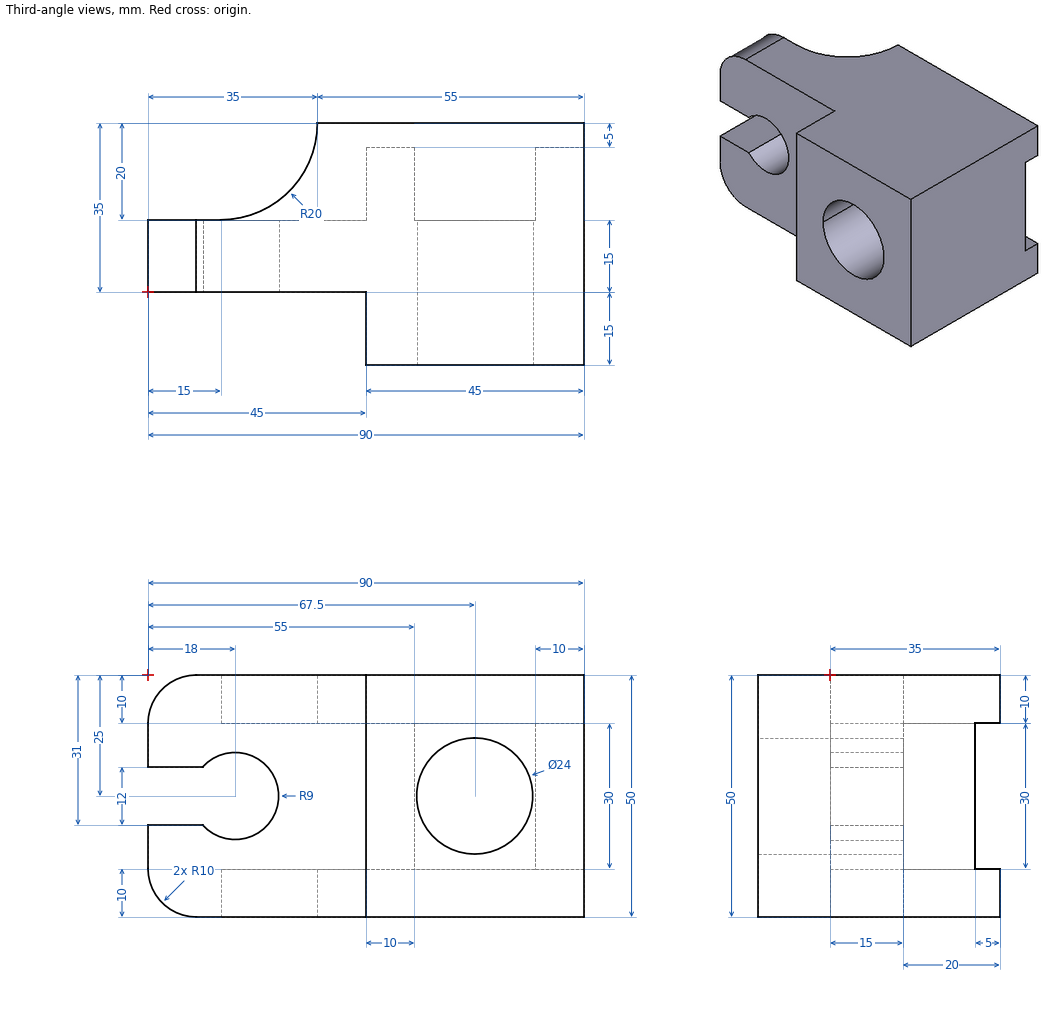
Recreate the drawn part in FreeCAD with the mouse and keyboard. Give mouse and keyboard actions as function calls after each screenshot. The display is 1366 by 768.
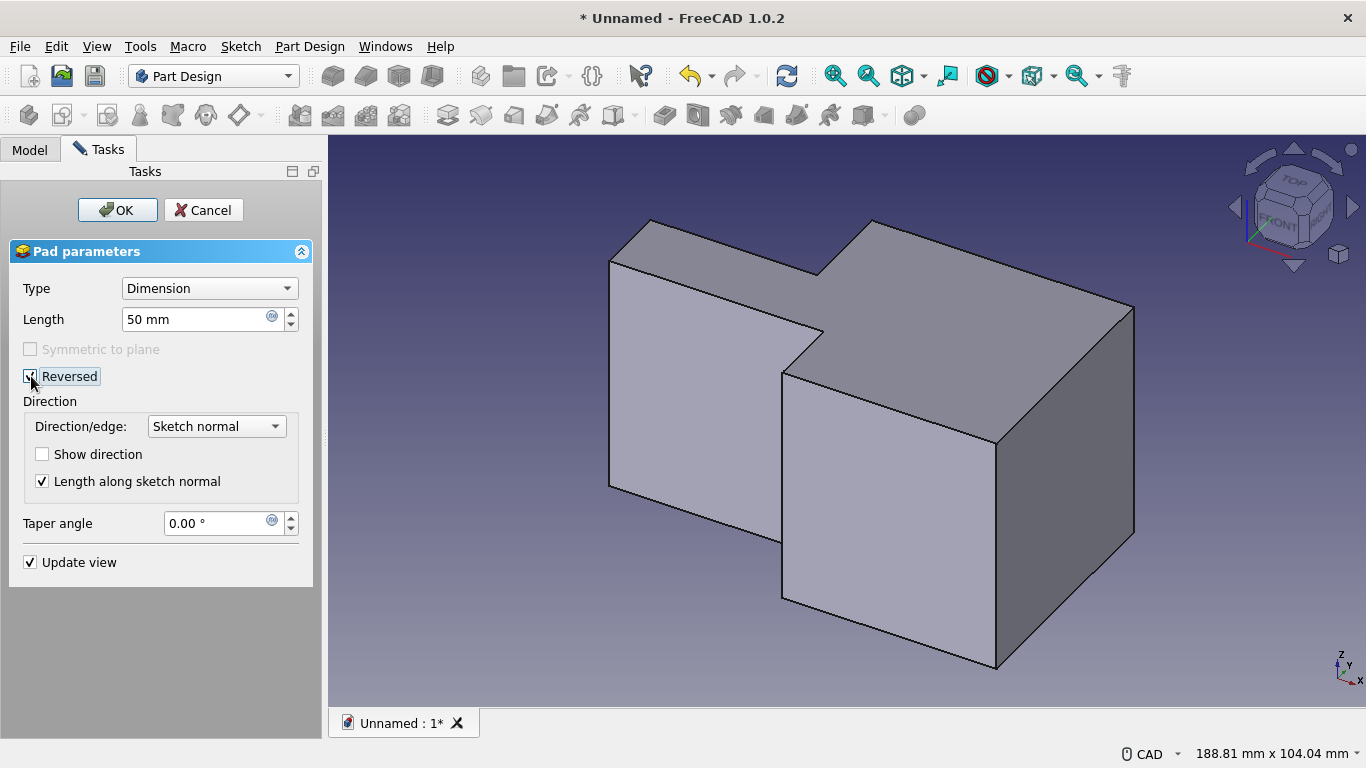
click(118, 210)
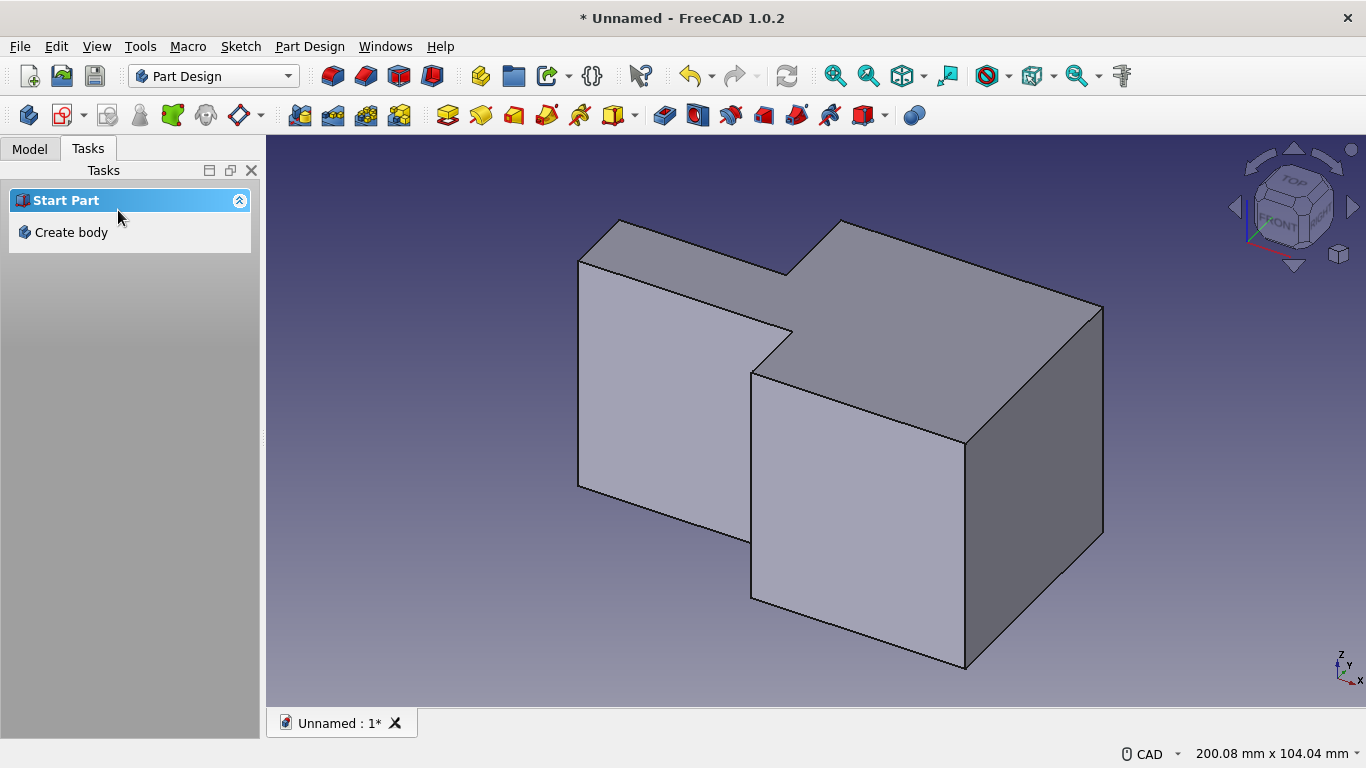
key(4)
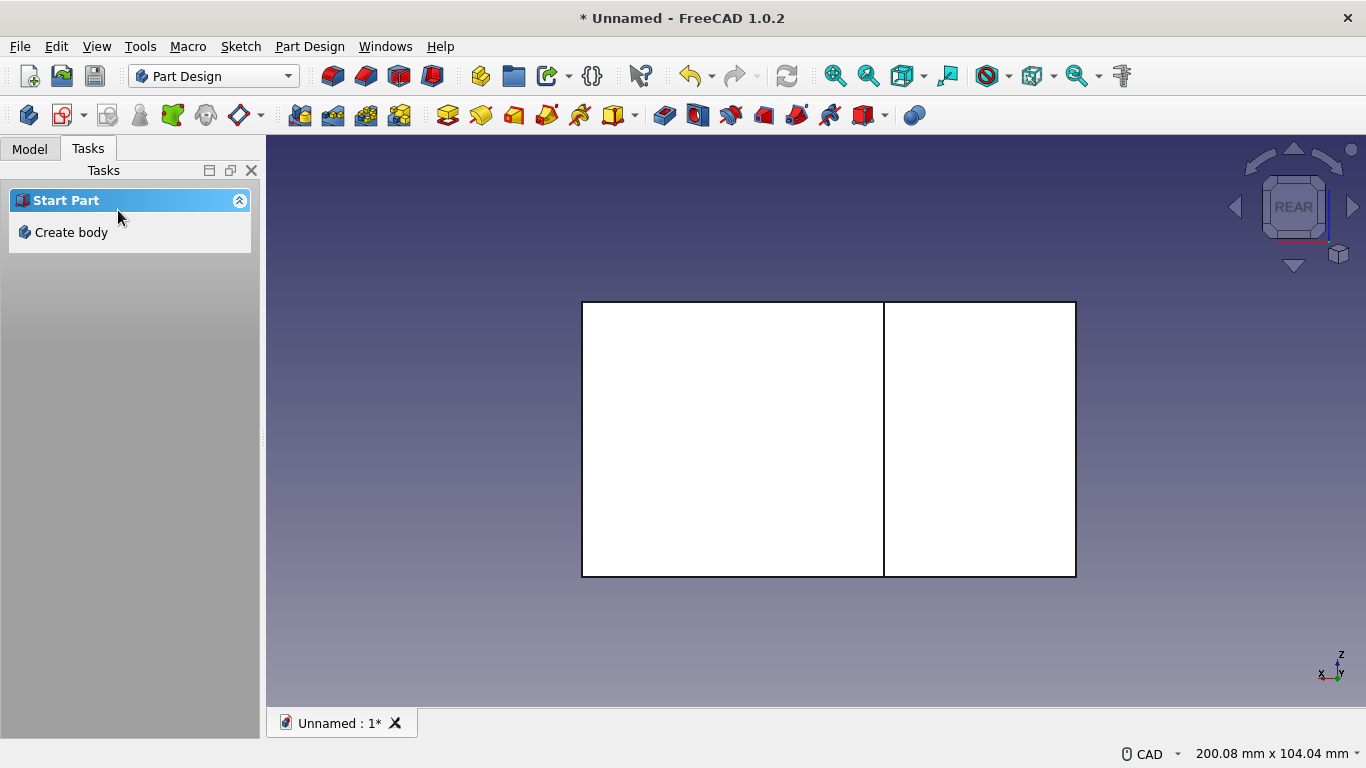
click(980, 399)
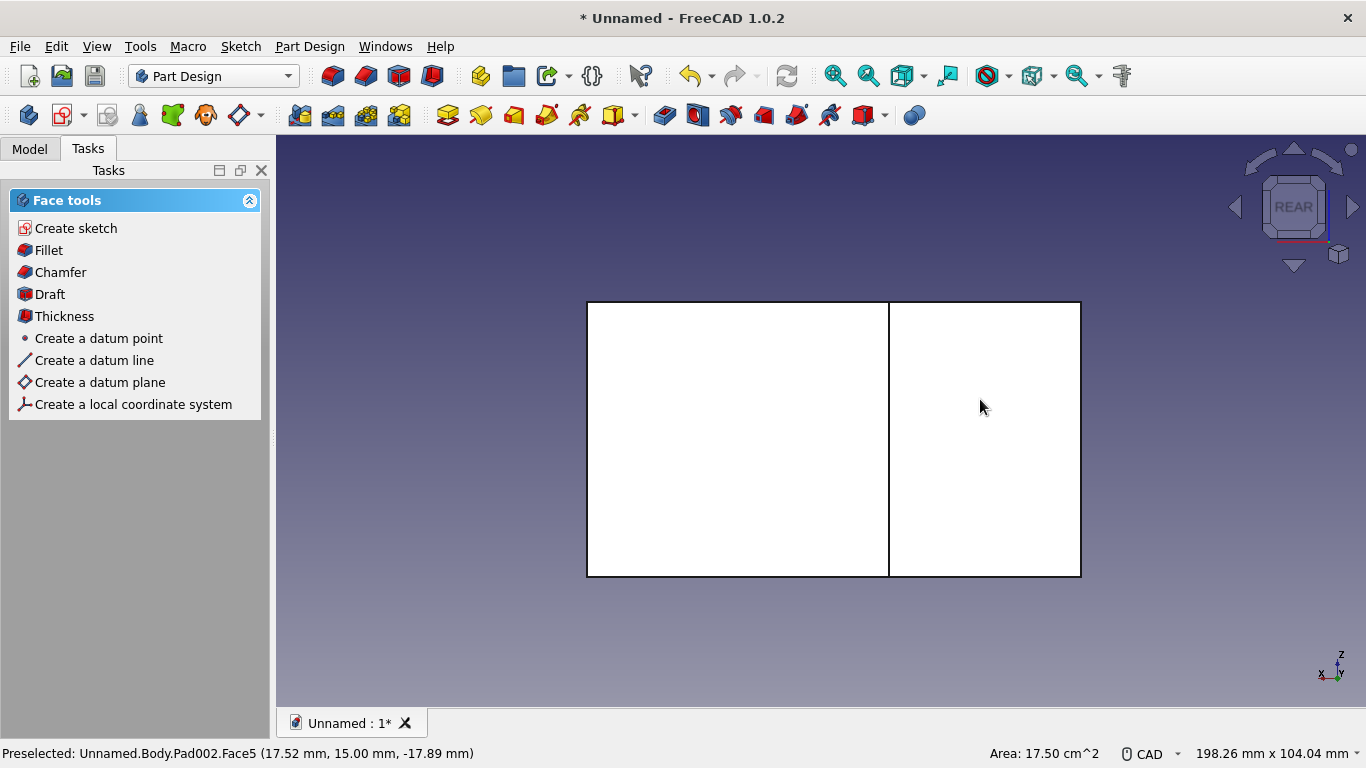
click(62, 116)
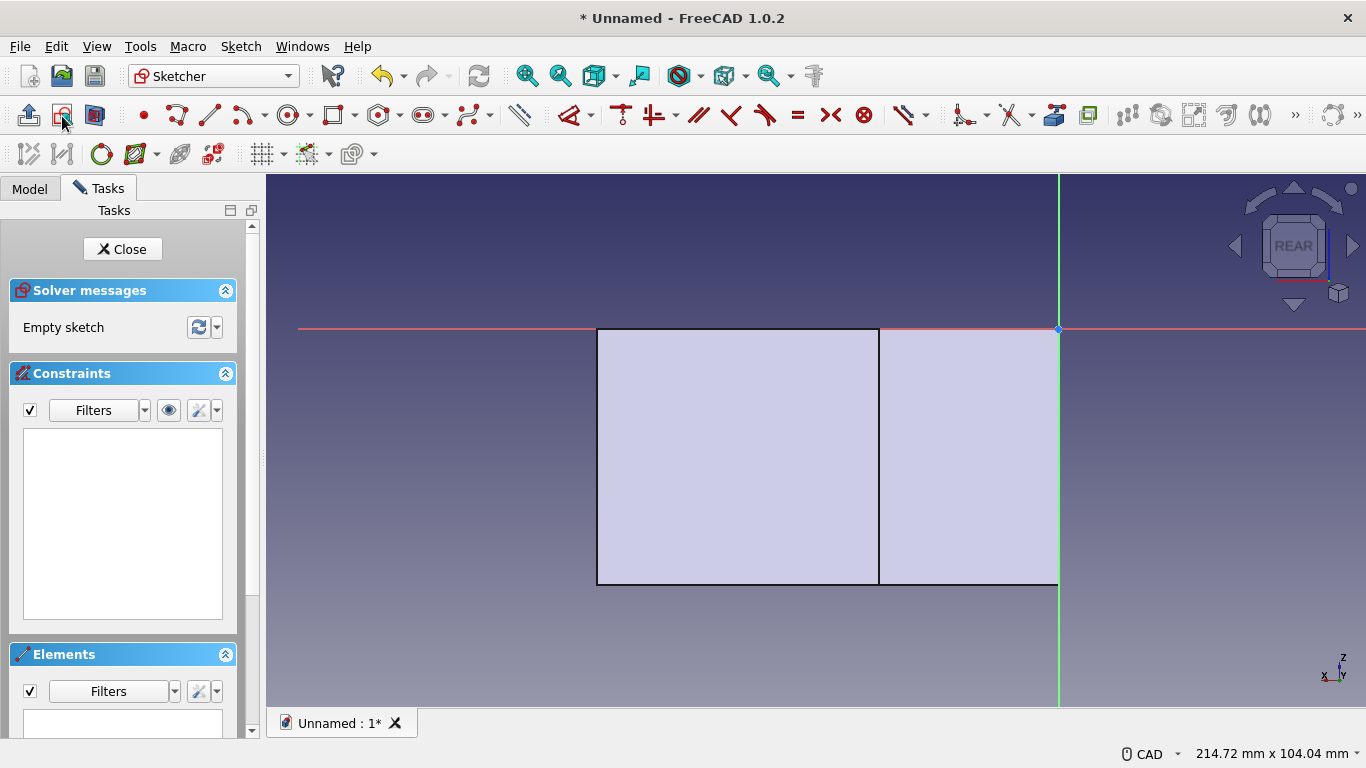
click(95, 116)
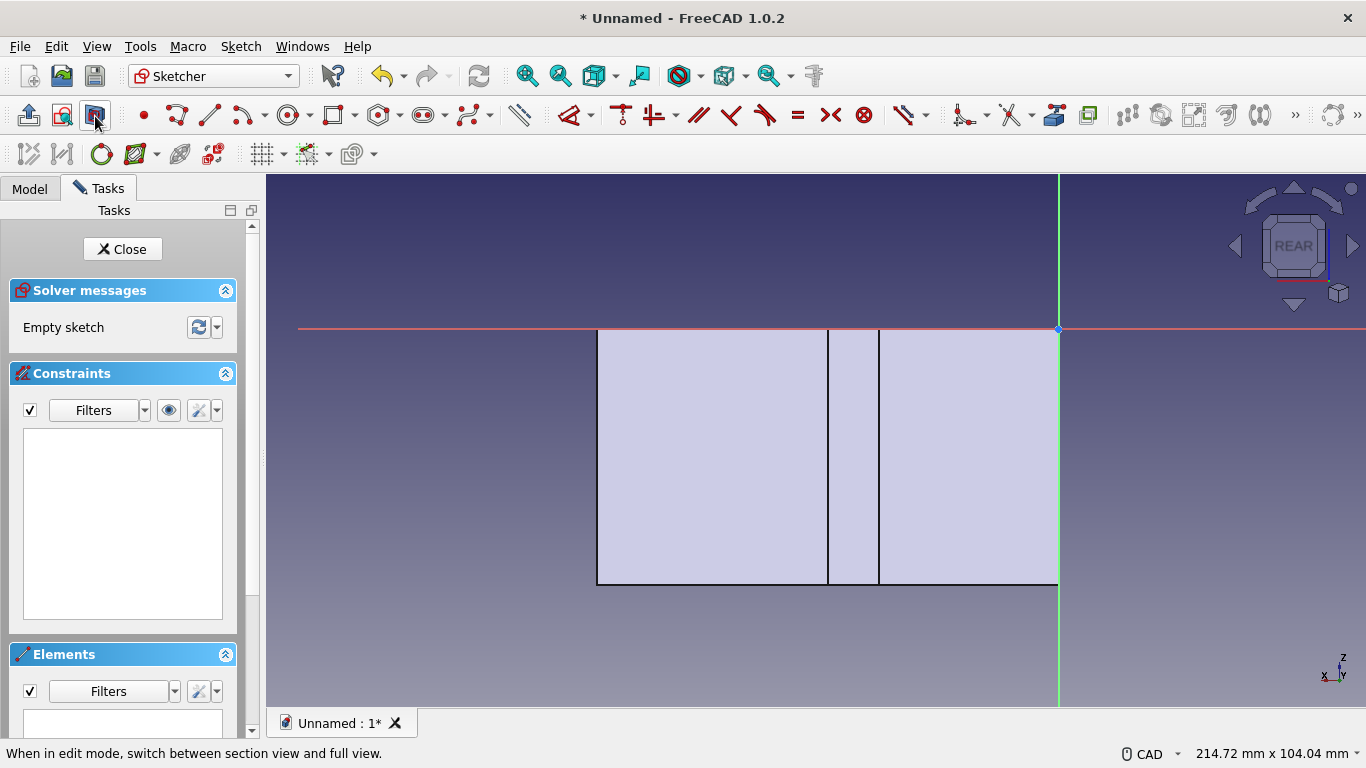
click(177, 116)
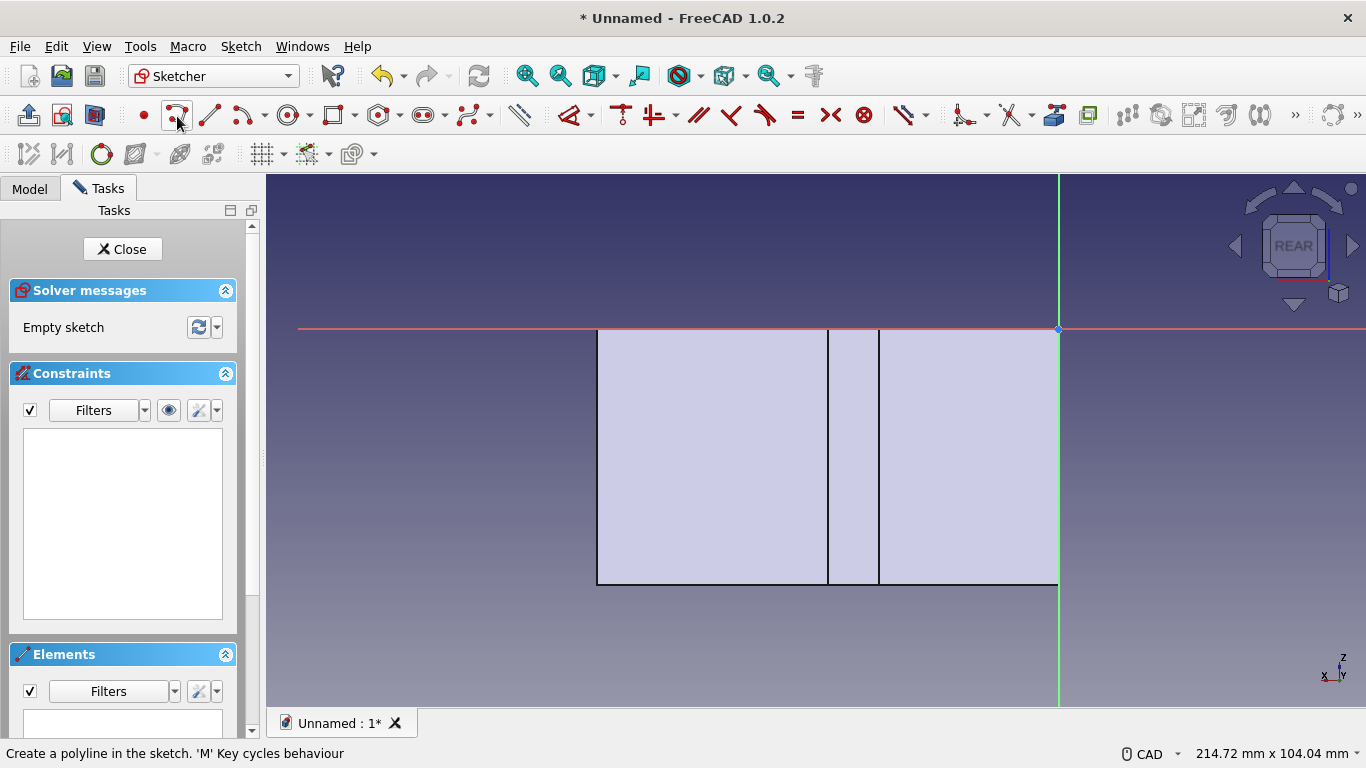
click(1007, 585)
click(1059, 585)
click(1050, 534)
right_click(1050, 534)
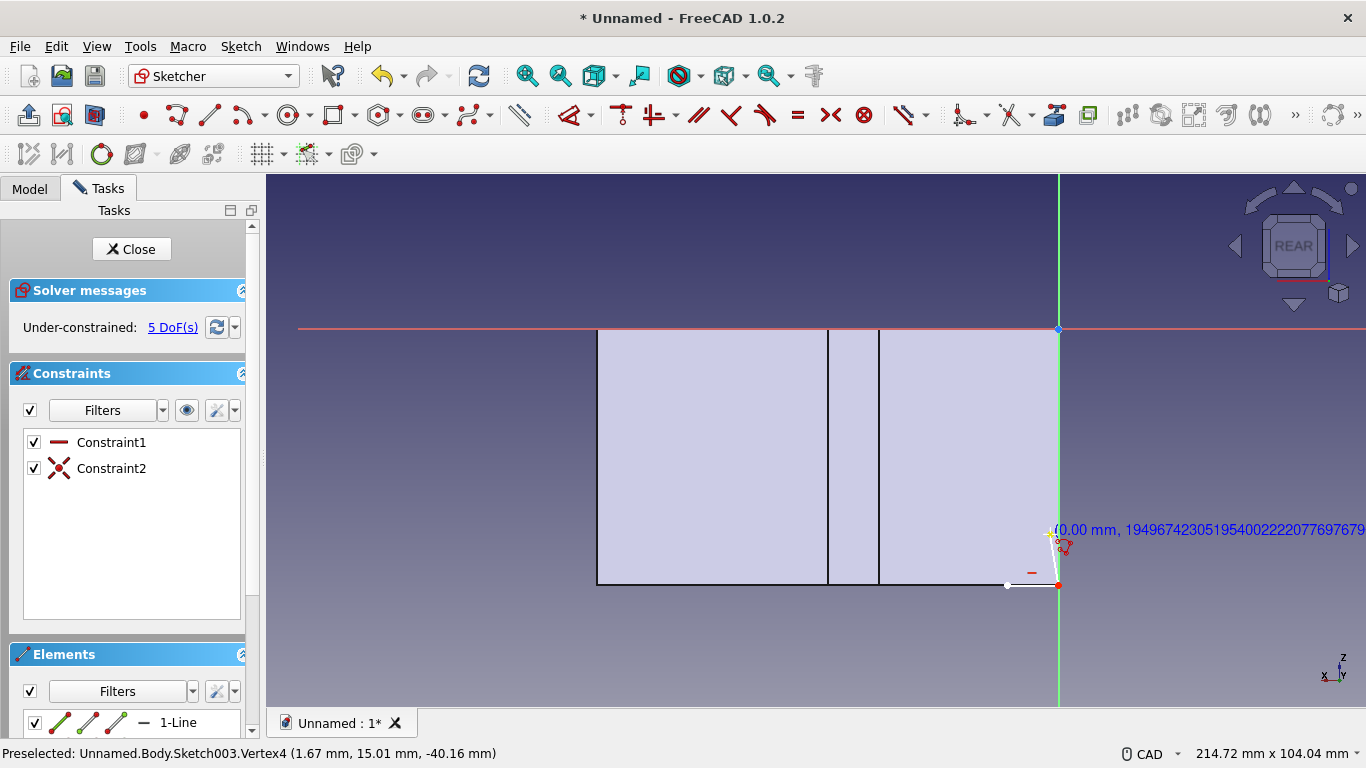
key(g)
key(3)
key(a)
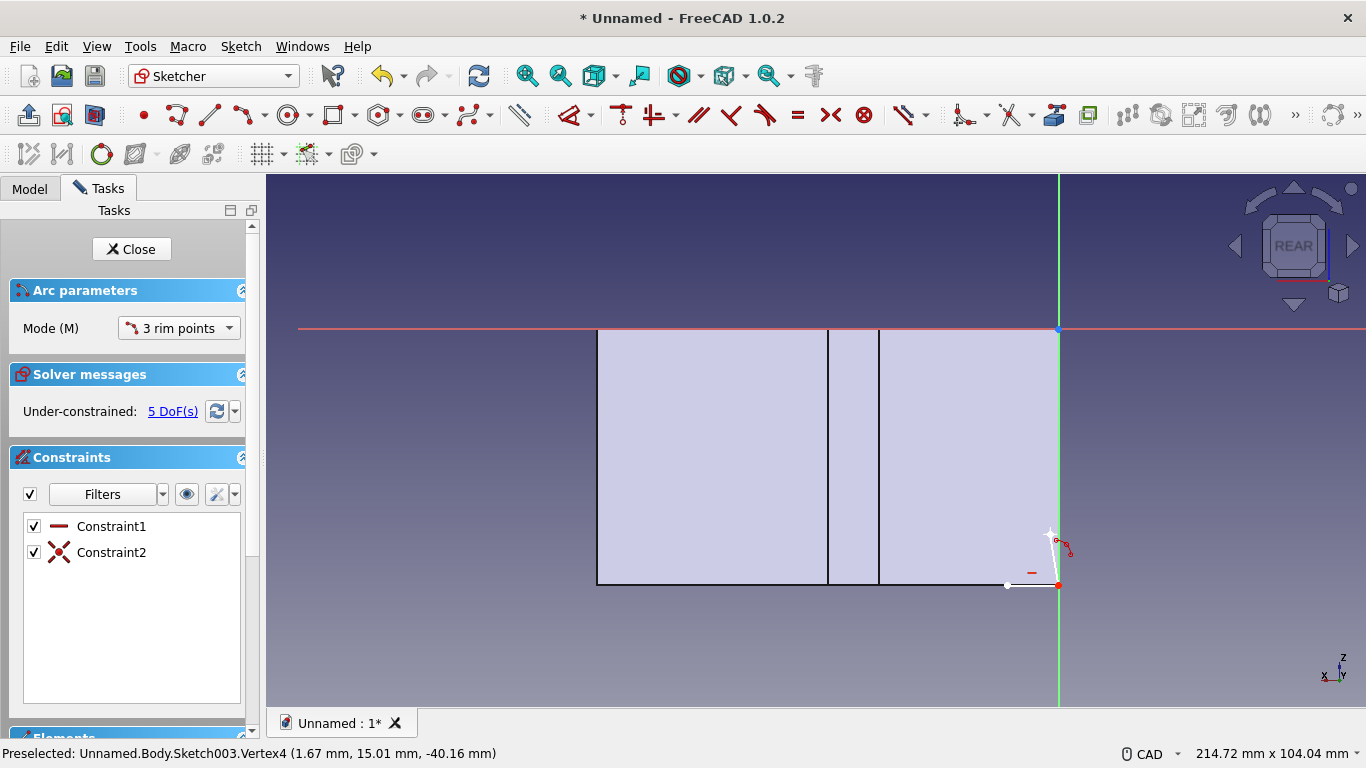
click(1050, 535)
click(1007, 586)
click(1044, 570)